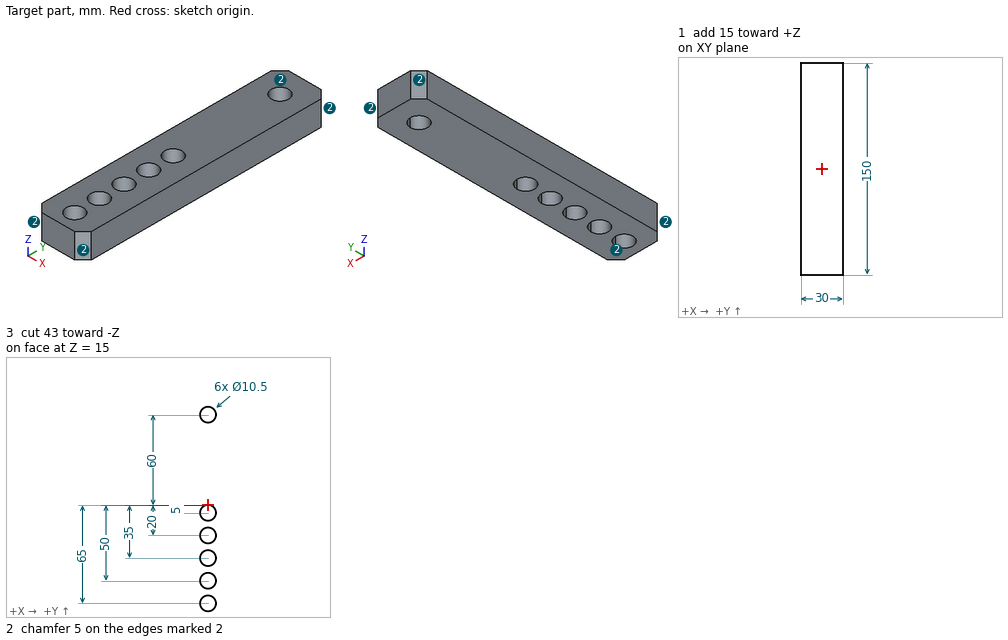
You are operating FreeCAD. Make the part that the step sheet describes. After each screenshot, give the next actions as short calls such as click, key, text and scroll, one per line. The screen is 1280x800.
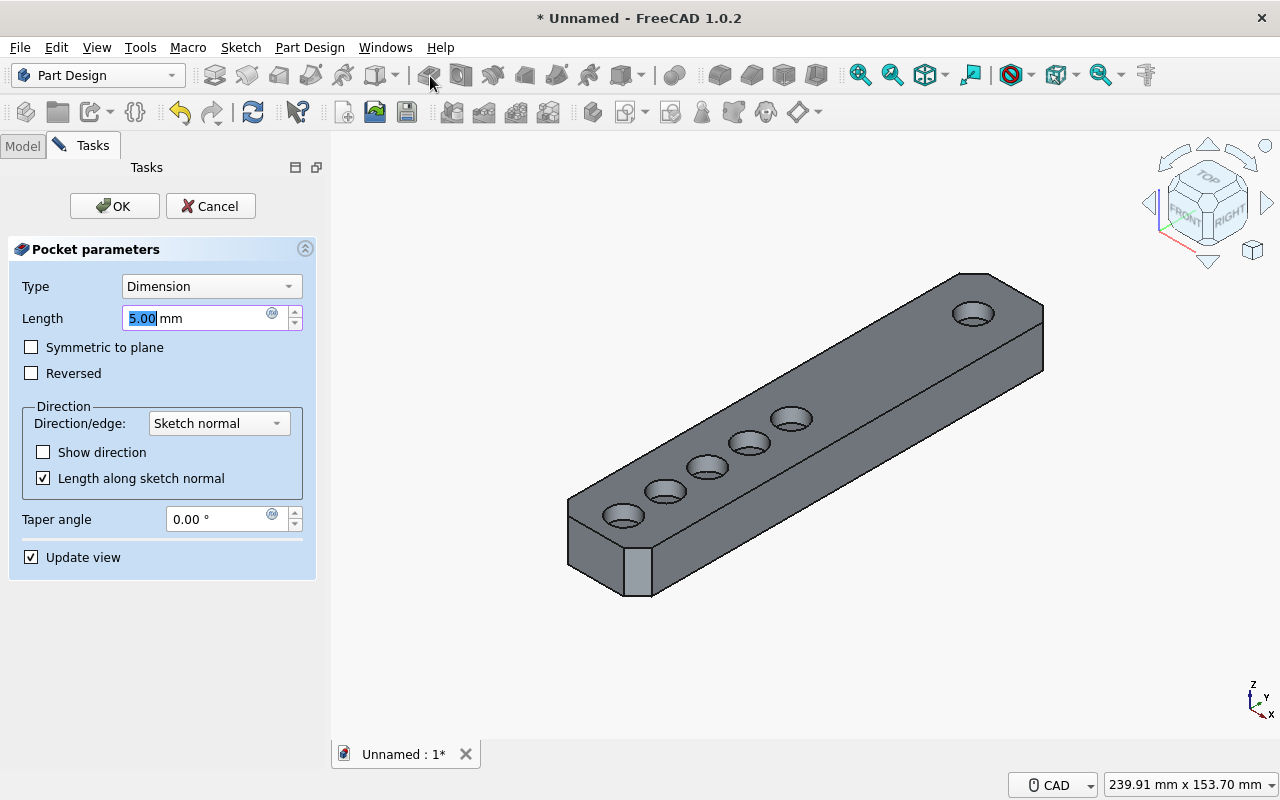
text(43)
key(Tab)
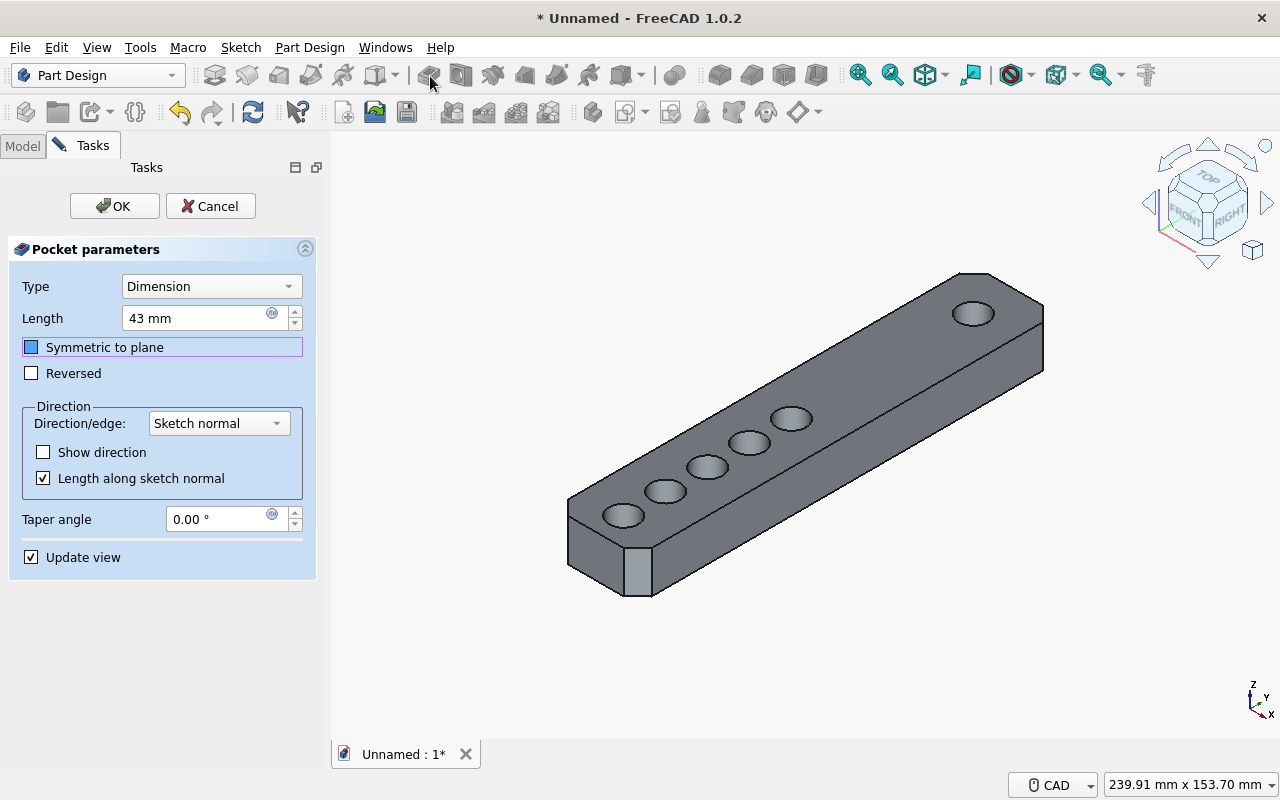
click(115, 206)